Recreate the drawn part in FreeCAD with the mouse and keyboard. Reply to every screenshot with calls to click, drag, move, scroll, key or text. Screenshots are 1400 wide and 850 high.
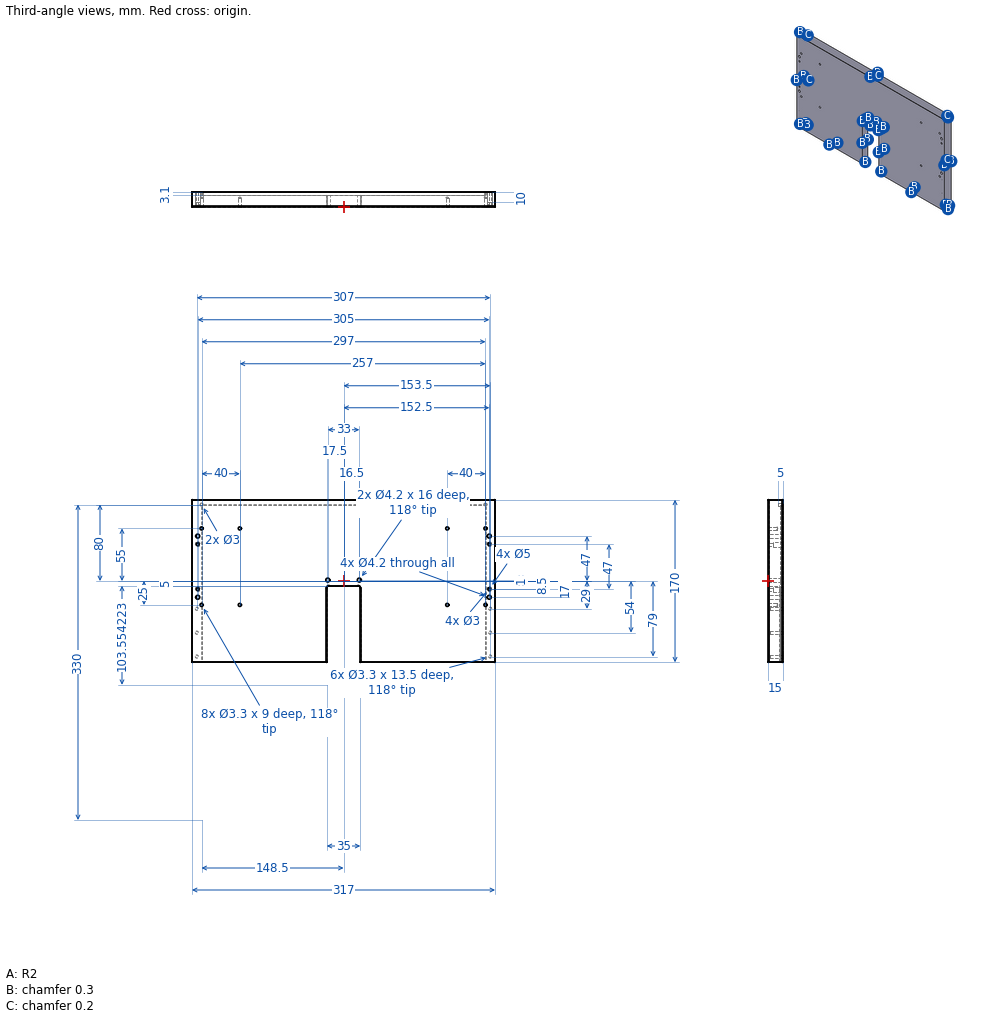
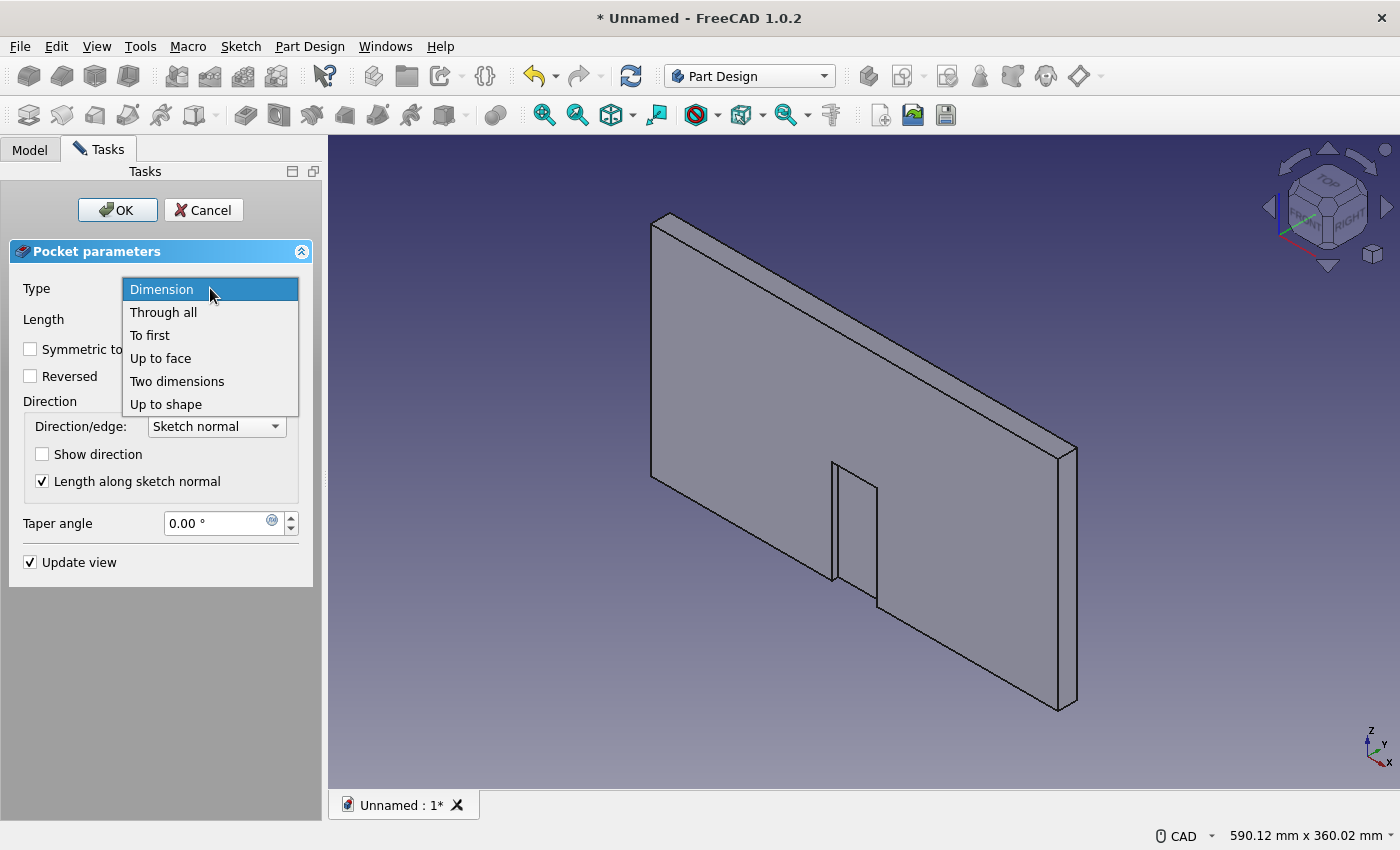
click(208, 312)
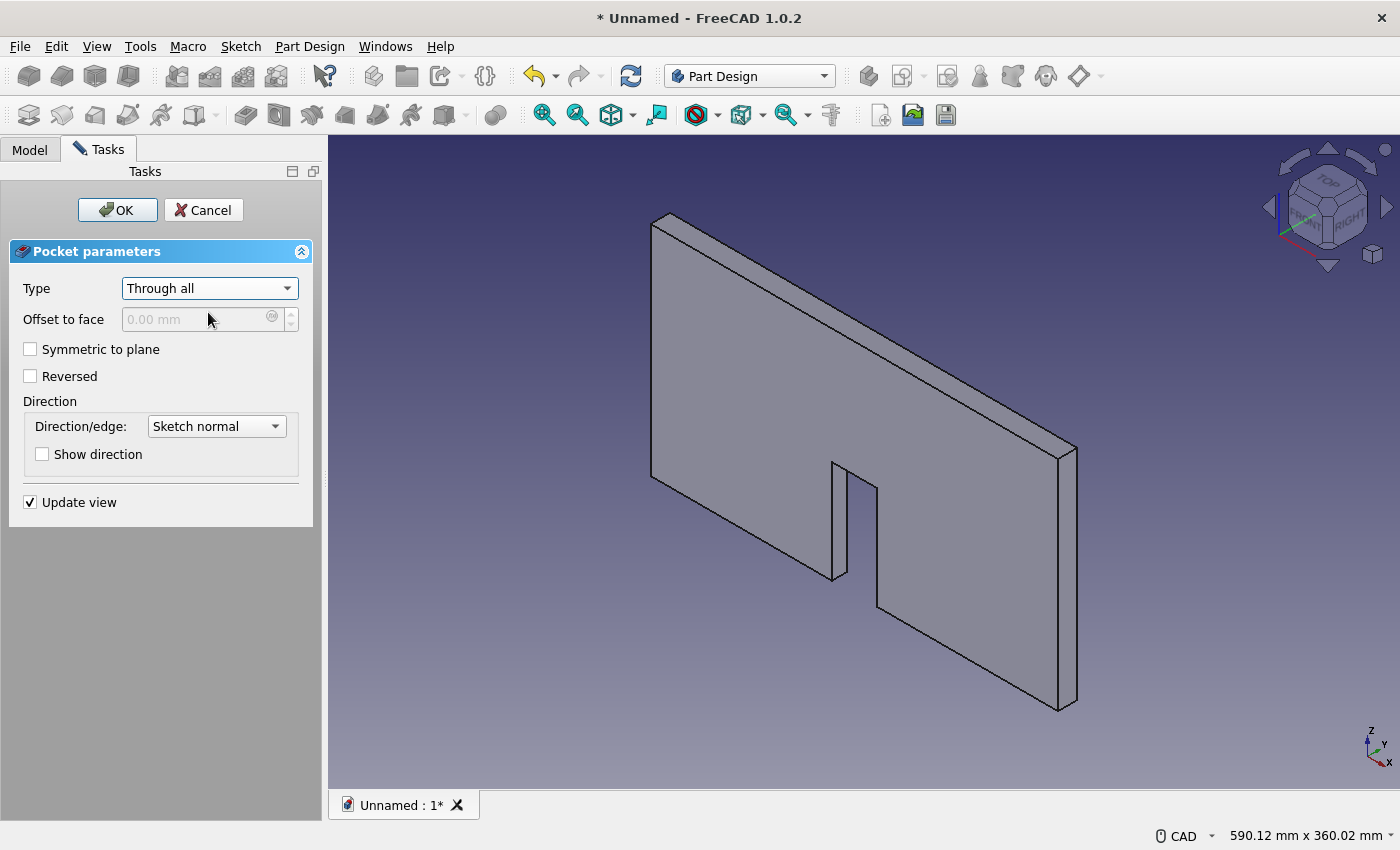
click(118, 210)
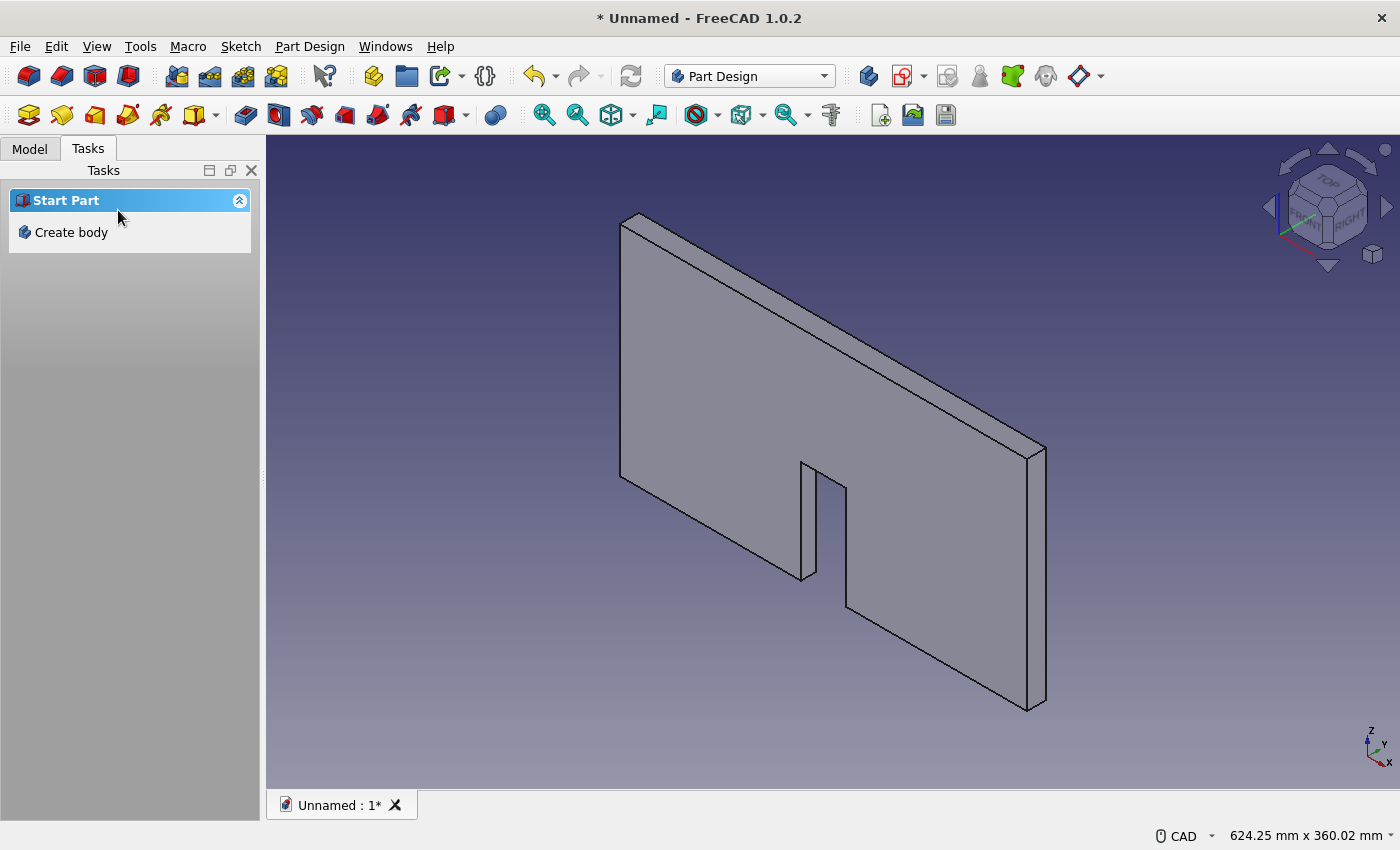
click(902, 76)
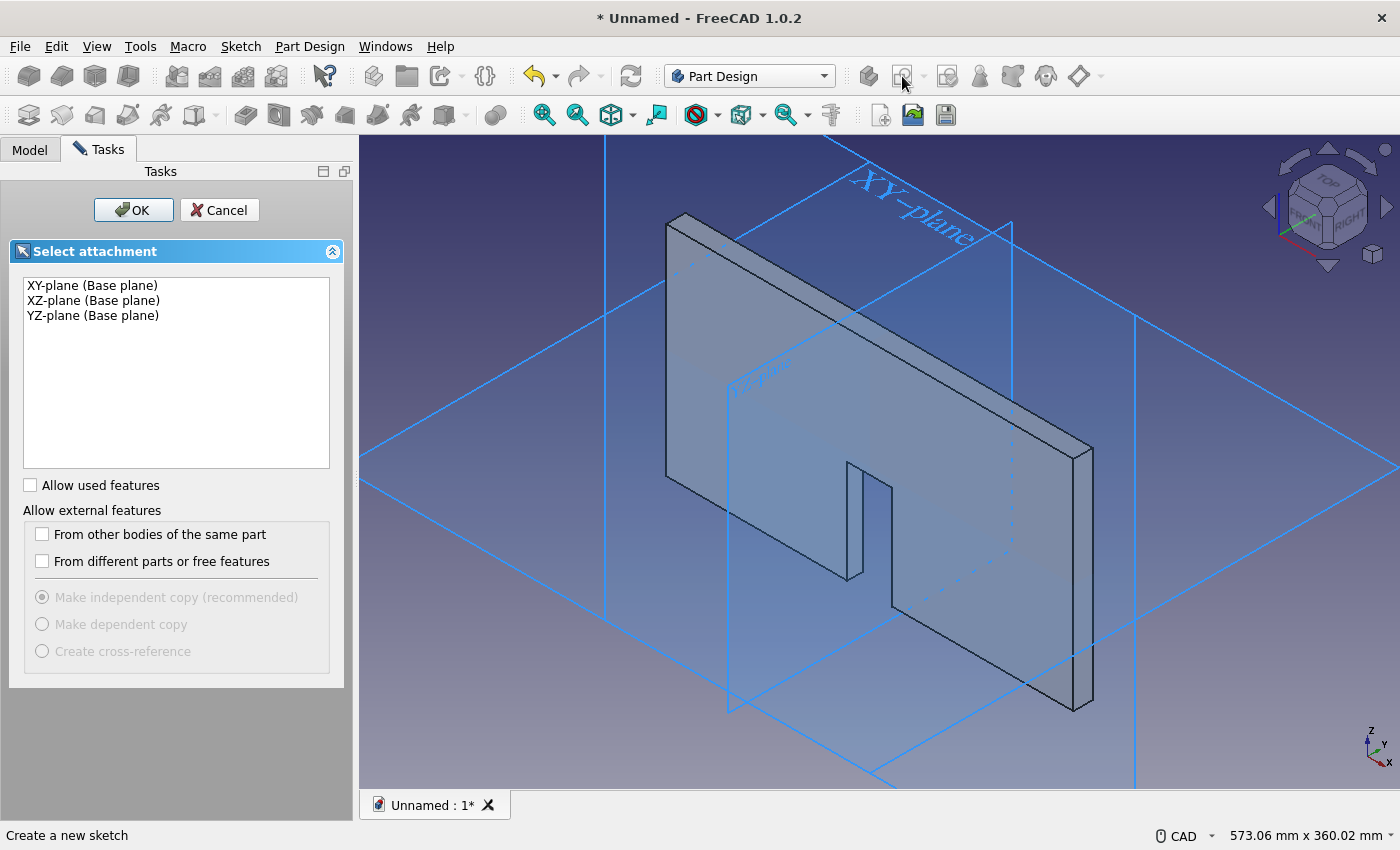
click(84, 300)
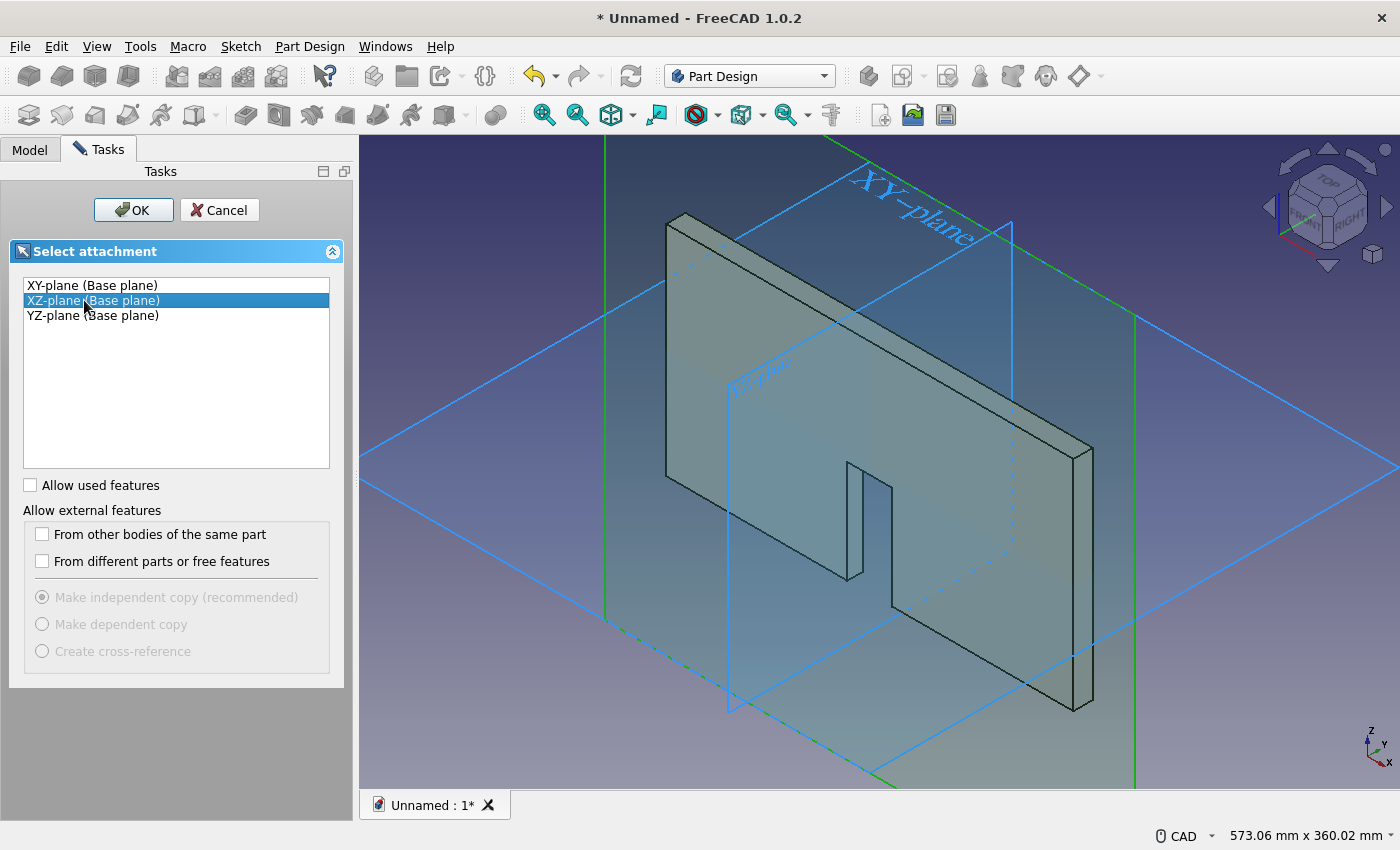
click(134, 210)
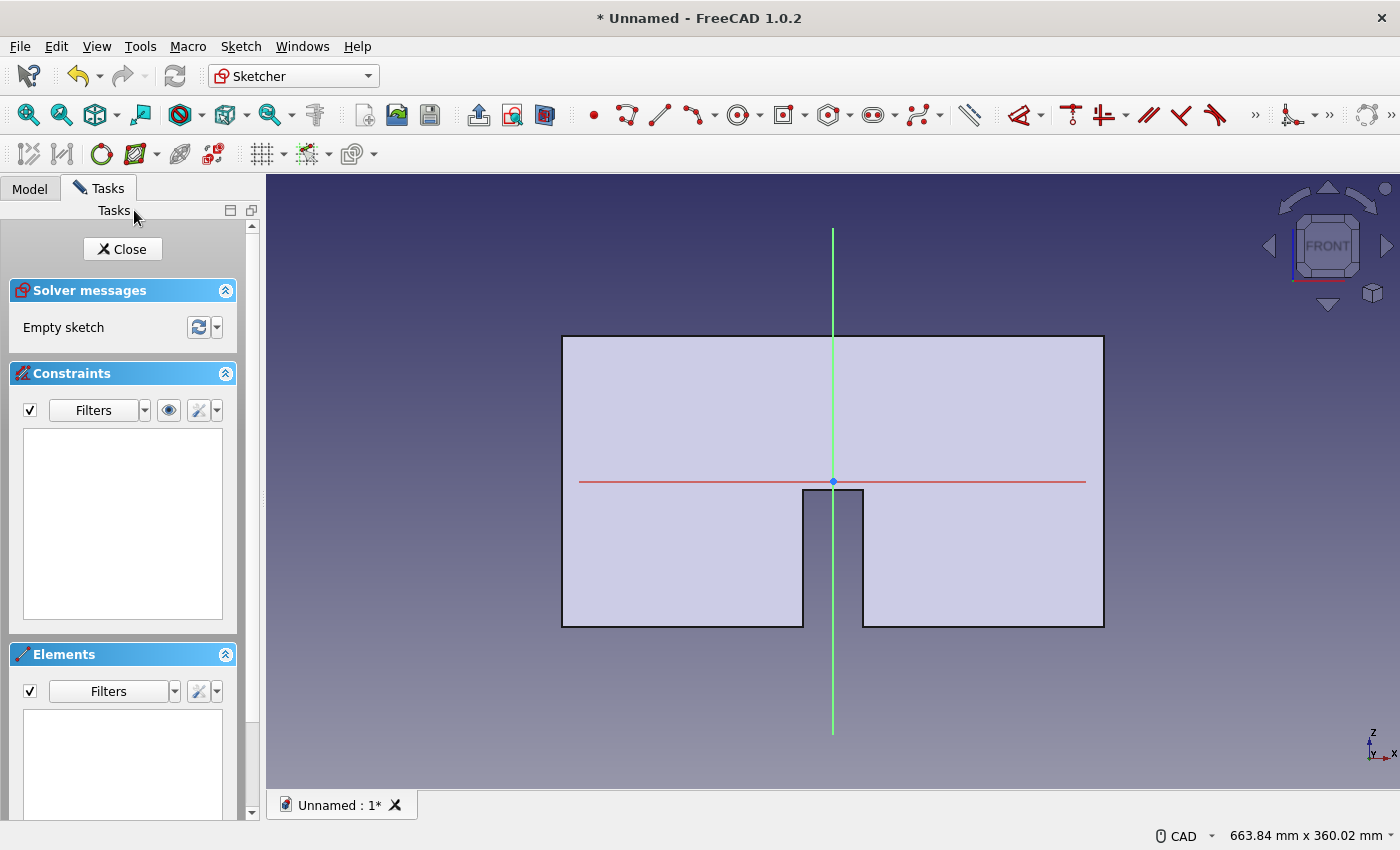
scroll(840, 480, up, 12)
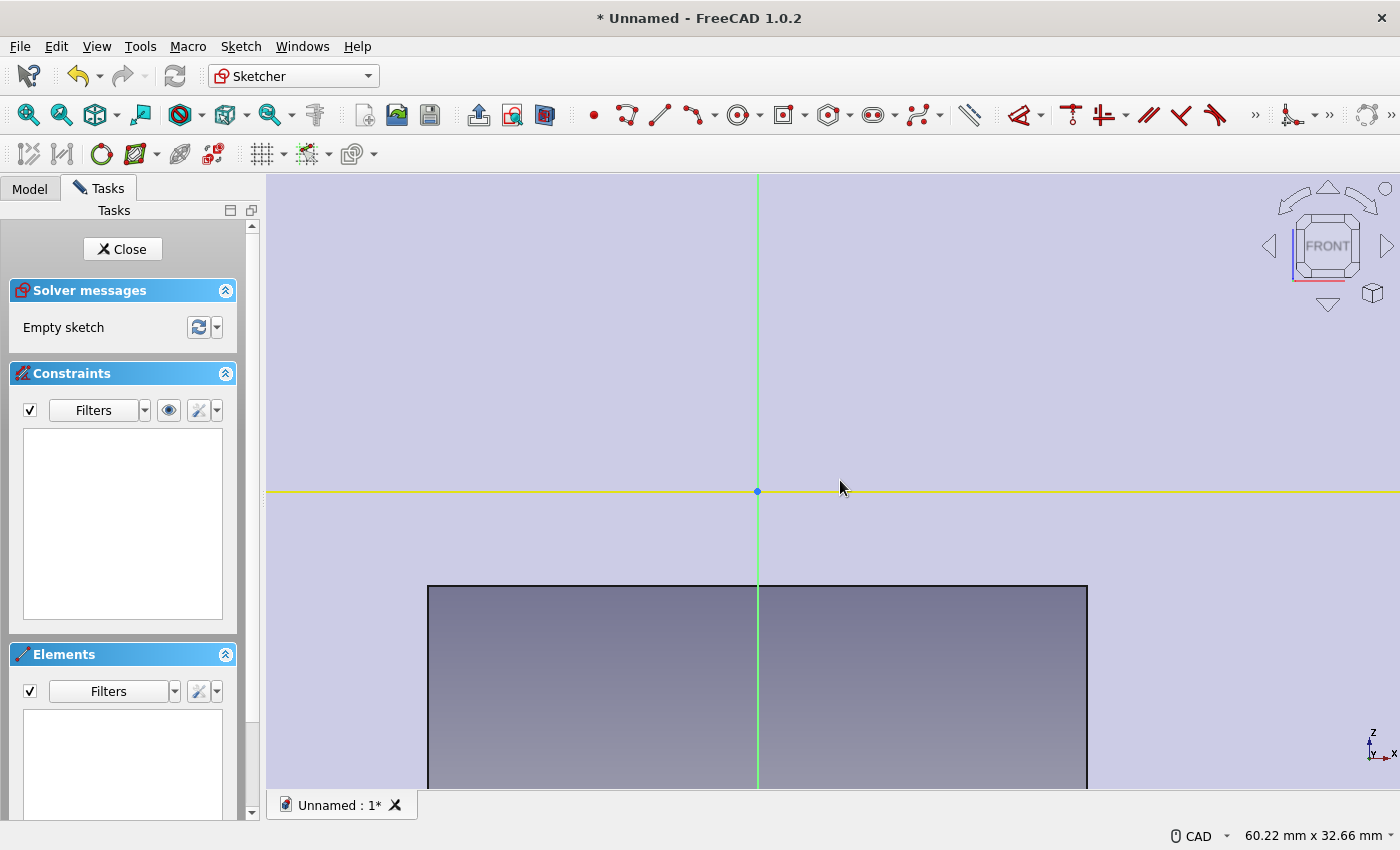
key(g)
key(c)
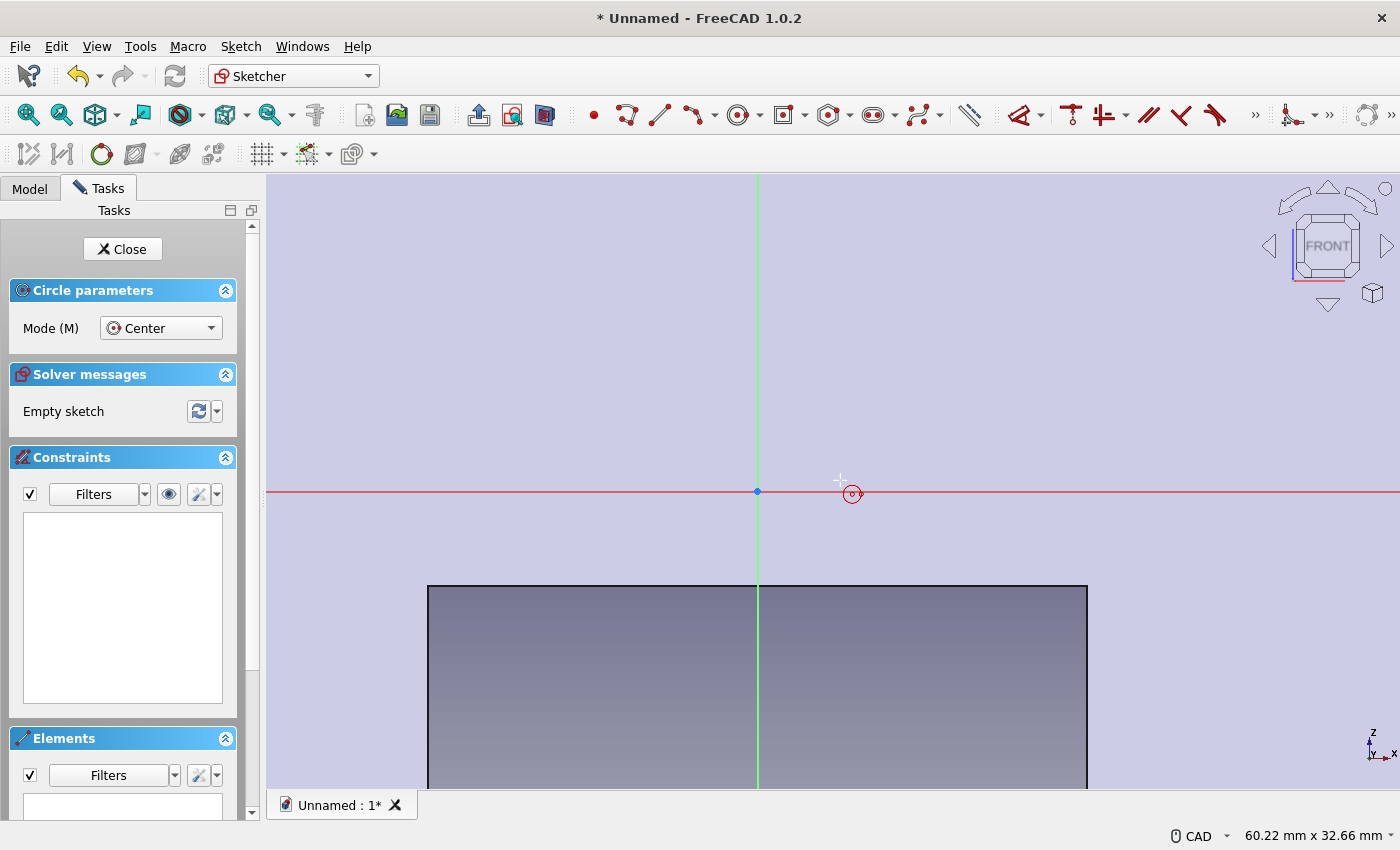
click(1068, 473)
click(1096, 445)